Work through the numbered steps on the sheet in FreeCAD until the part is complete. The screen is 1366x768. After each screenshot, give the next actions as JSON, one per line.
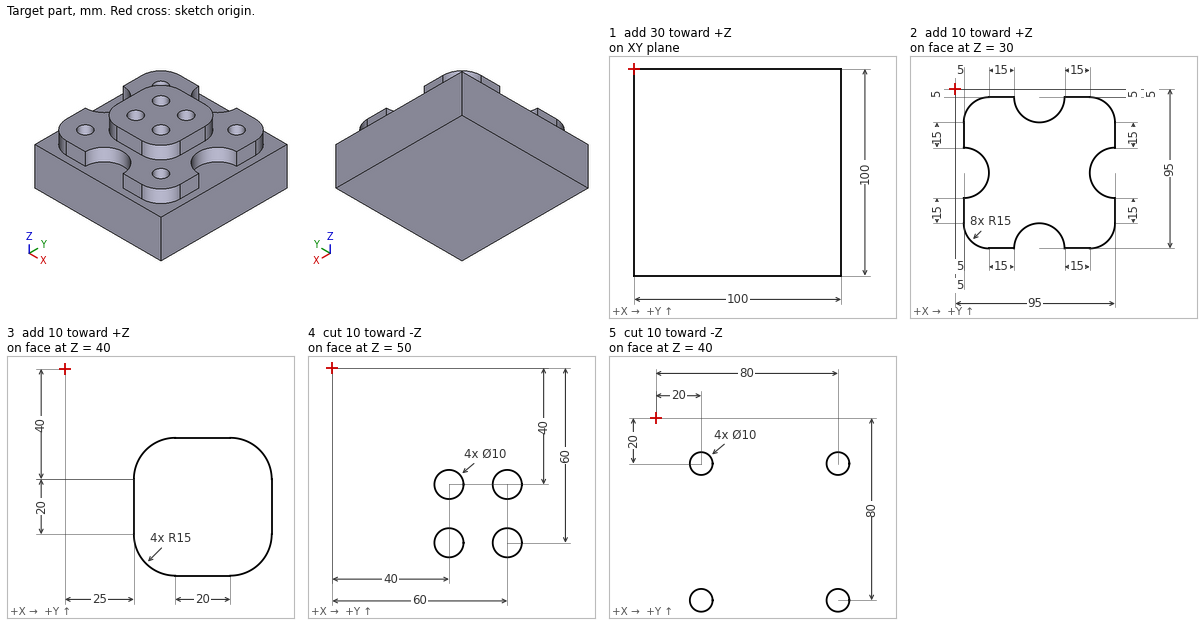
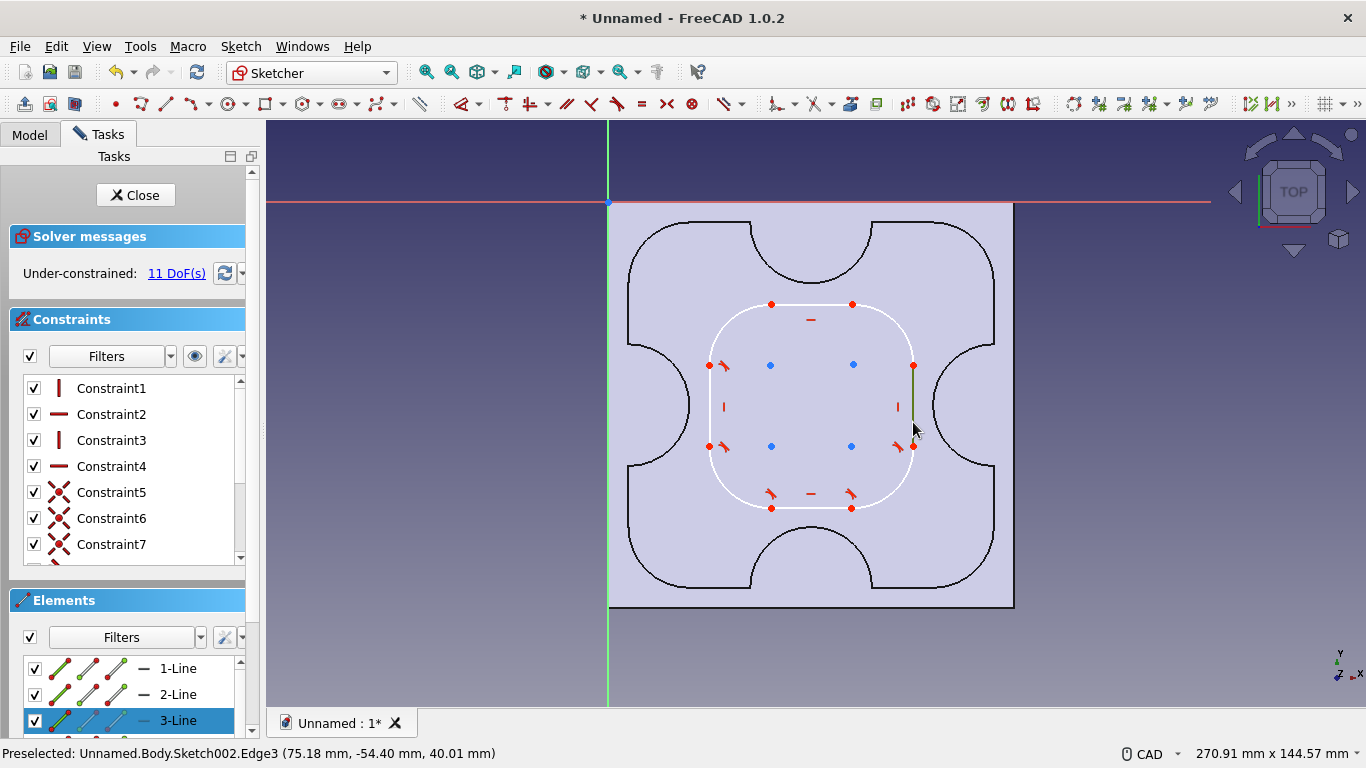
{"action": "left_click", "coordinate": [907, 338]}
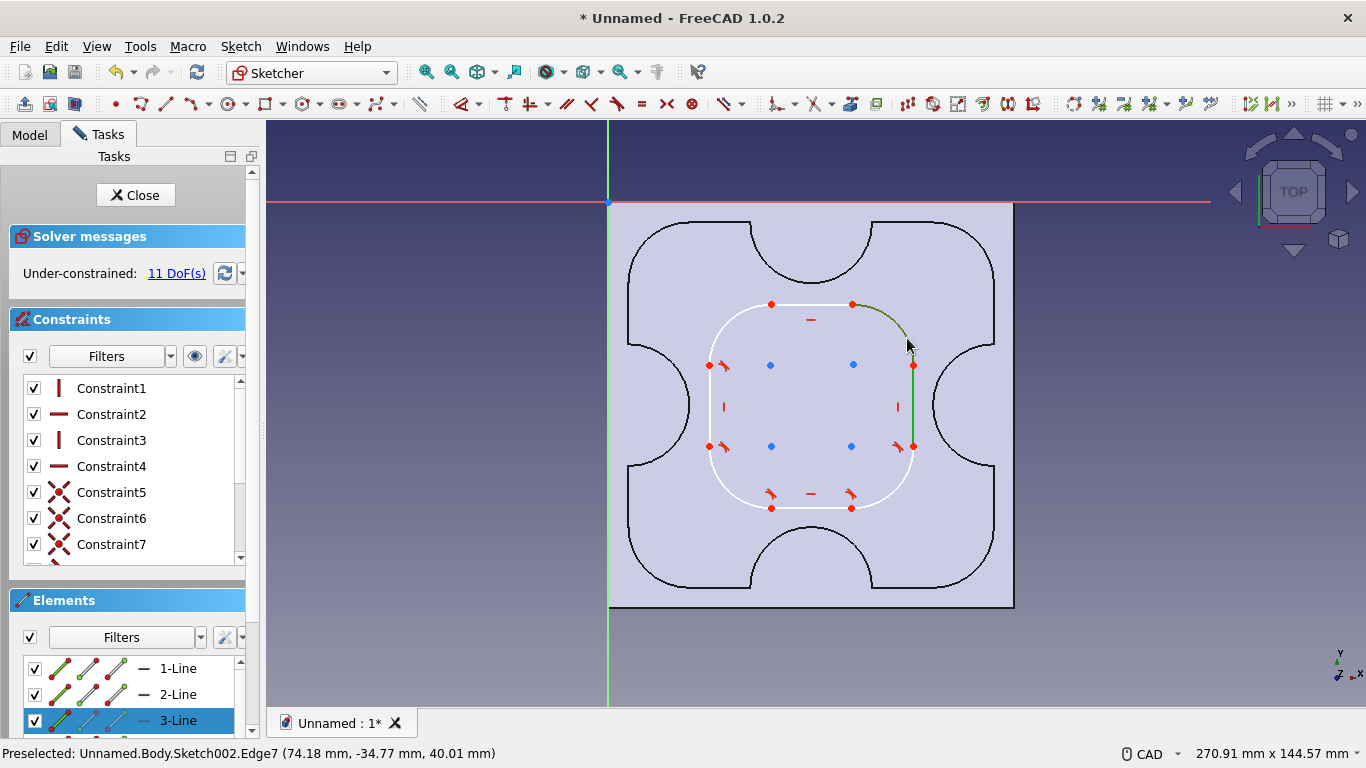
{"action": "key", "text": "t"}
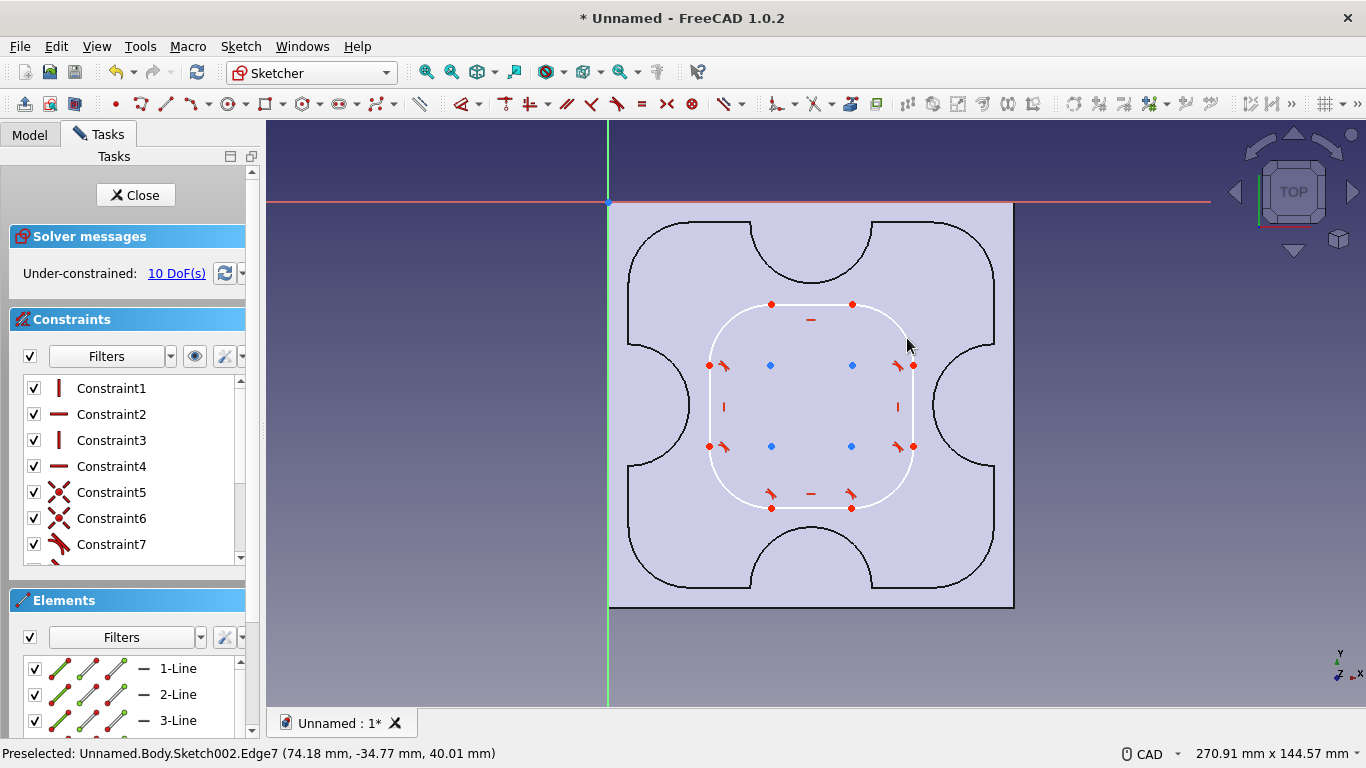
{"action": "left_click", "coordinate": [828, 305]}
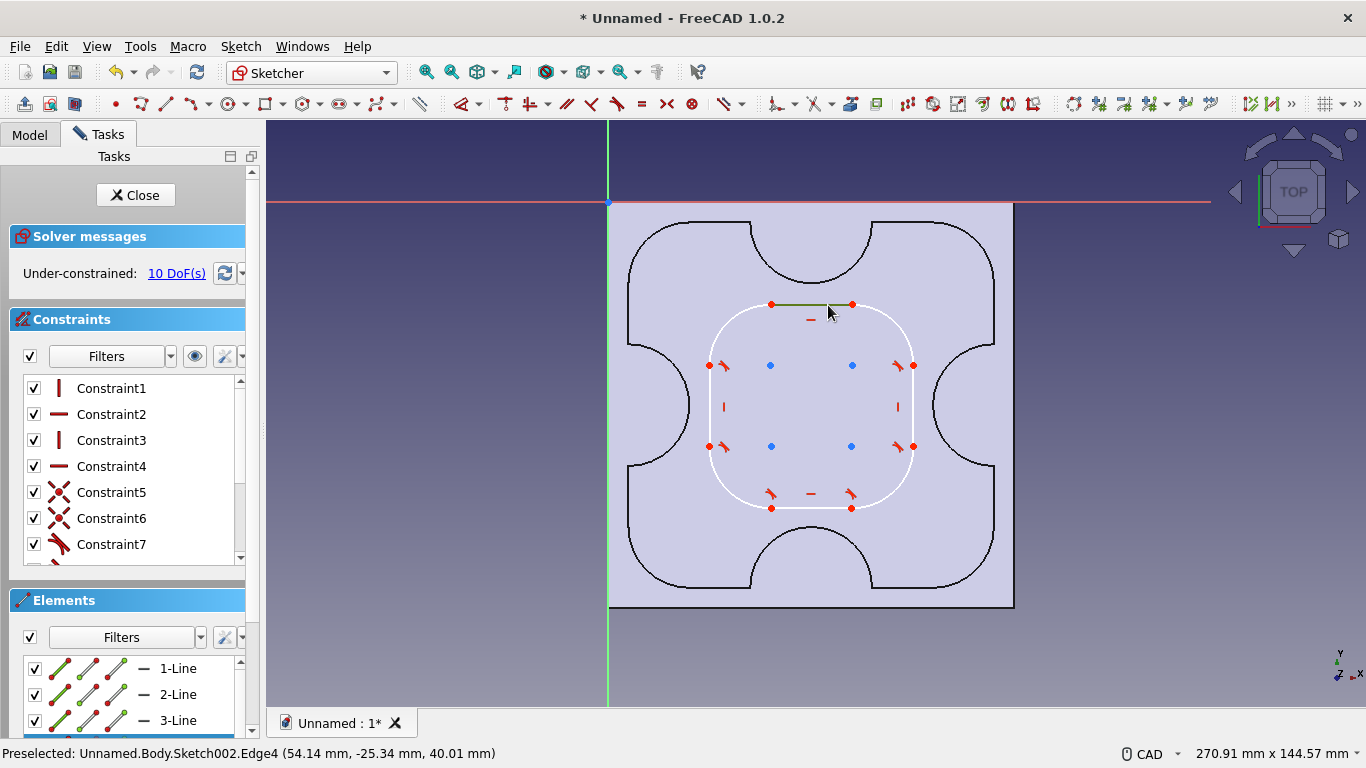
{"action": "left_click", "coordinate": [907, 338]}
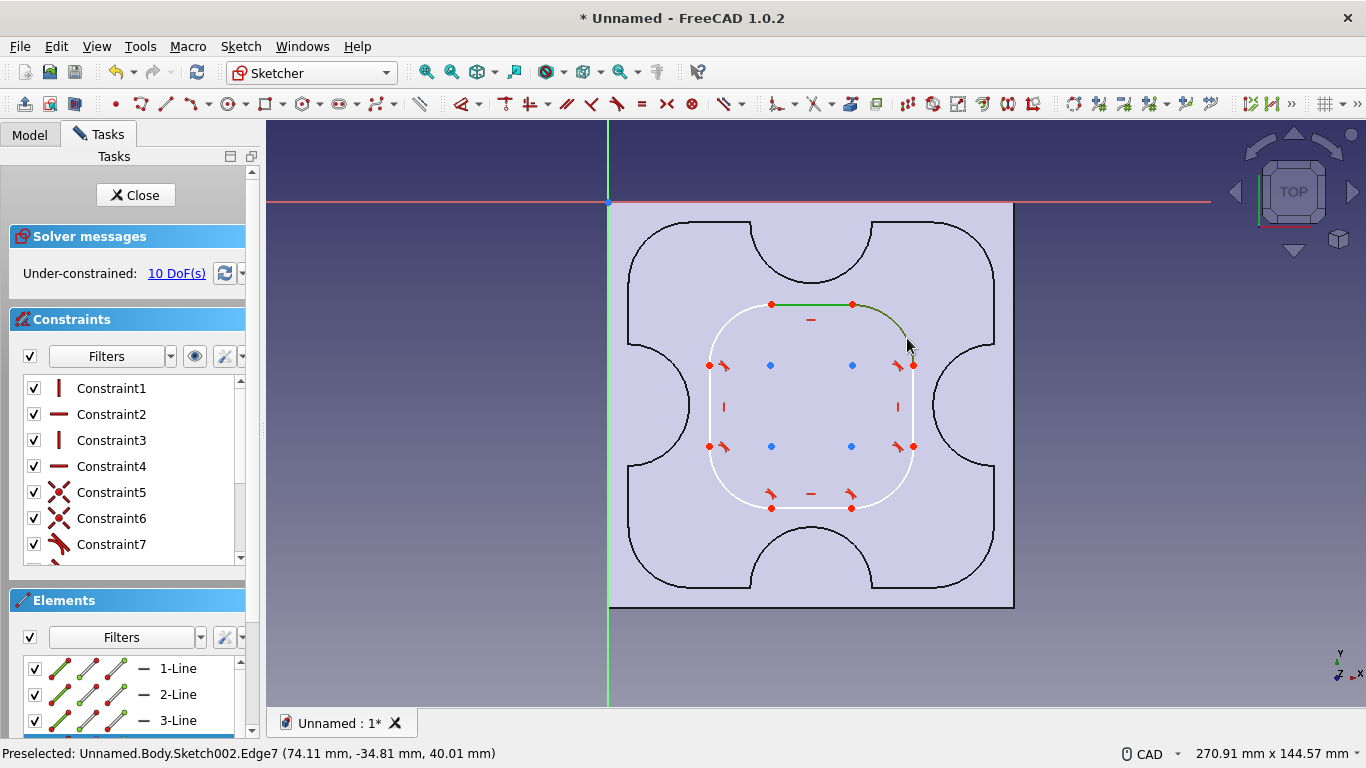
{"action": "left_click", "coordinate": [617, 104]}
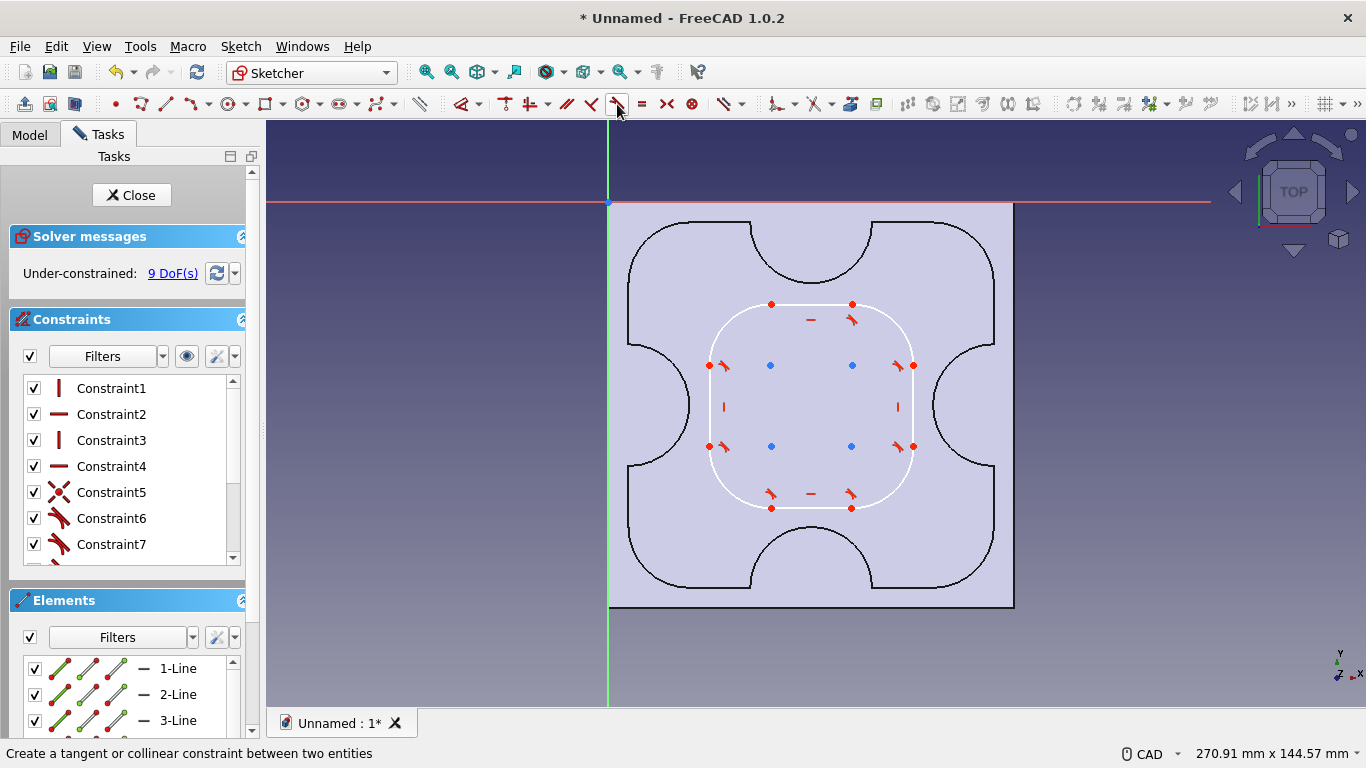
{"action": "left_click", "coordinate": [828, 305]}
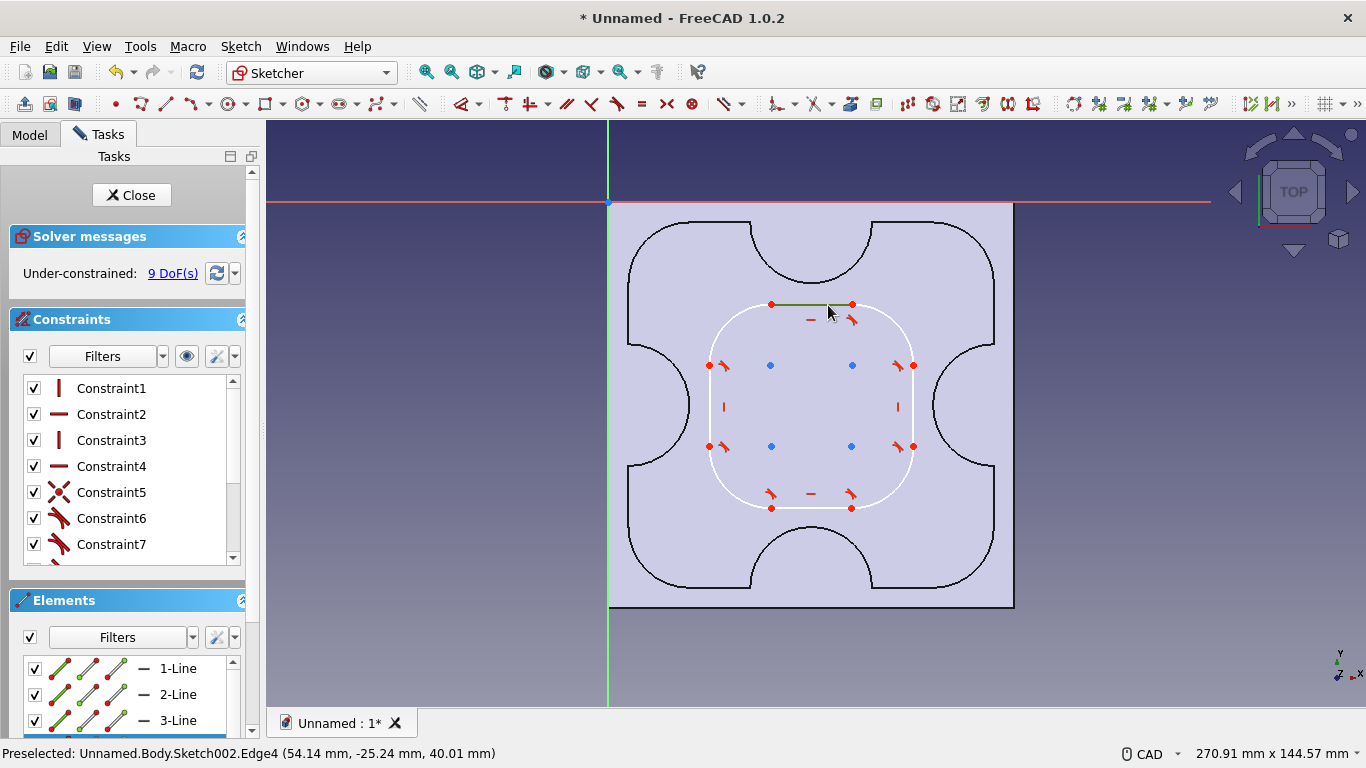
{"action": "left_click", "coordinate": [743, 311]}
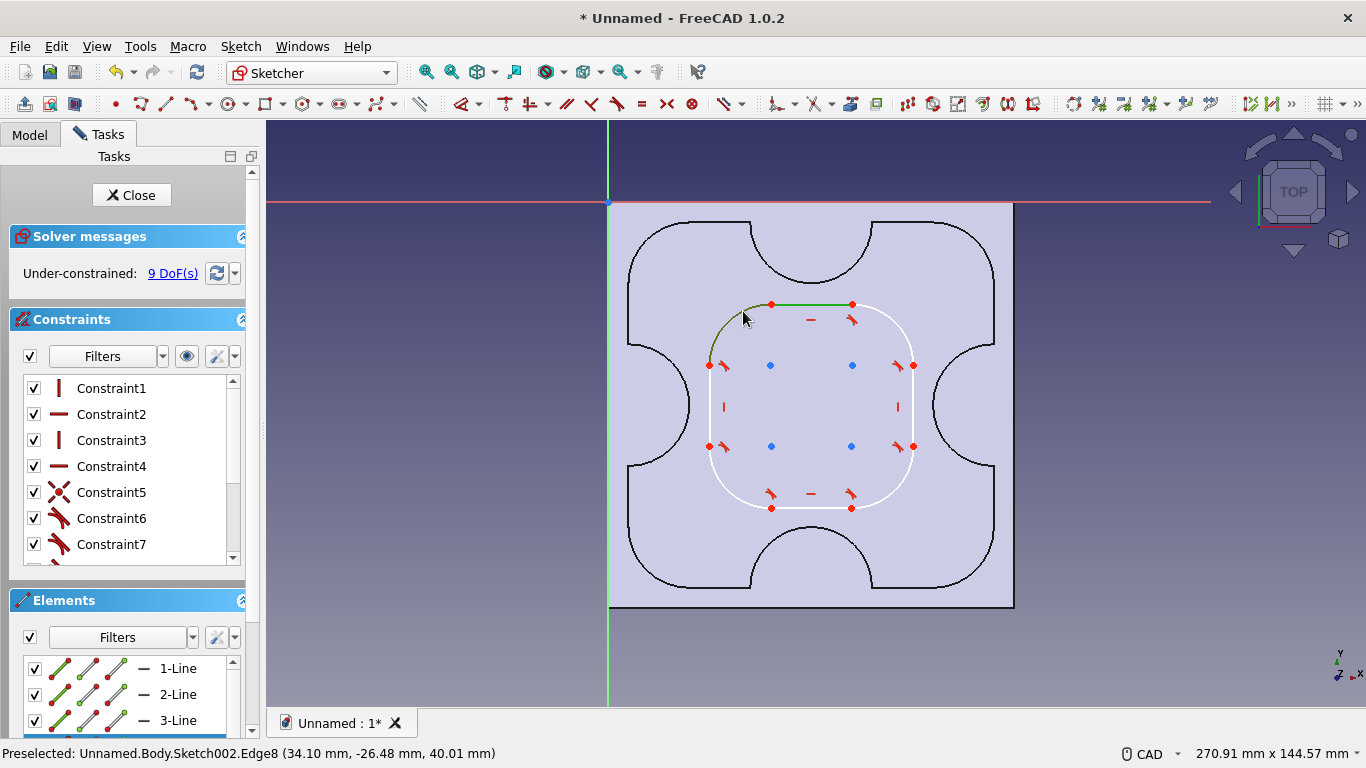
{"action": "left_click", "coordinate": [617, 104]}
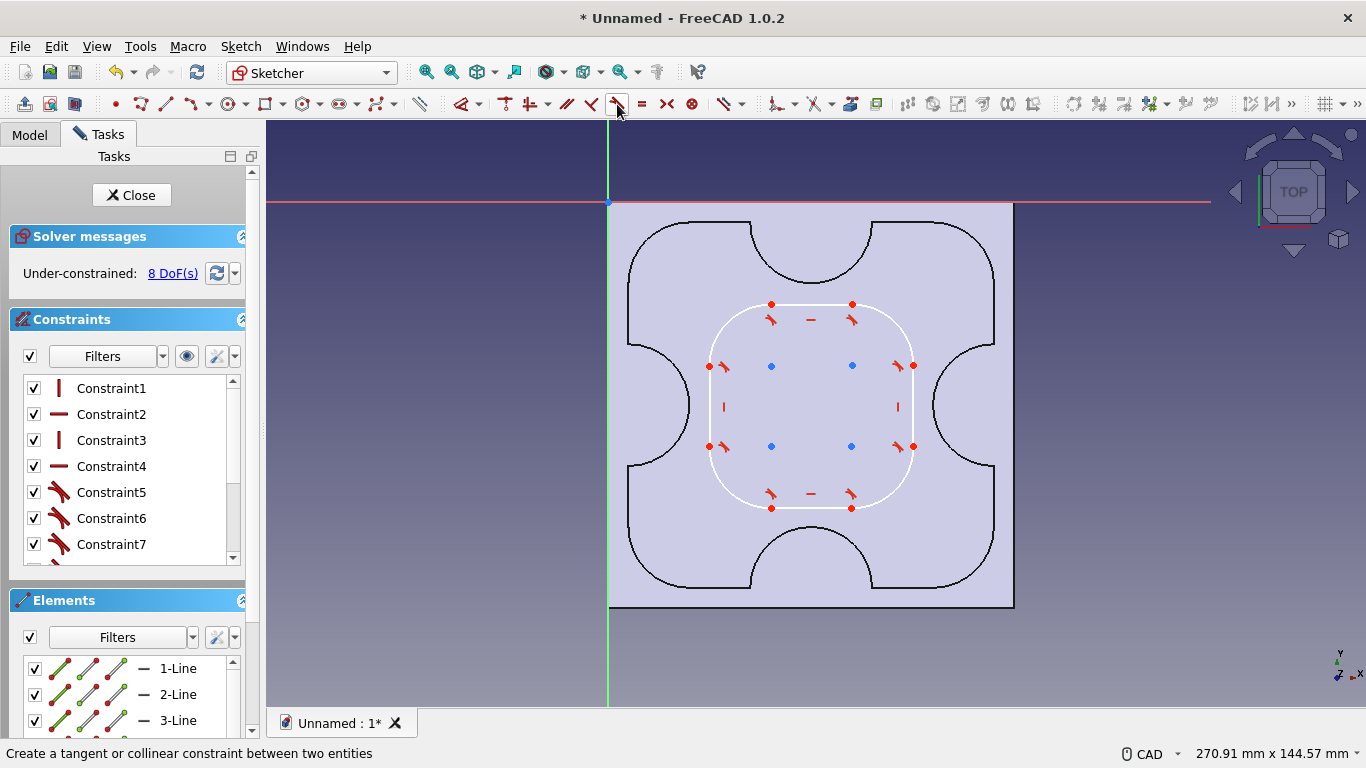
{"action": "left_click", "coordinate": [716, 475]}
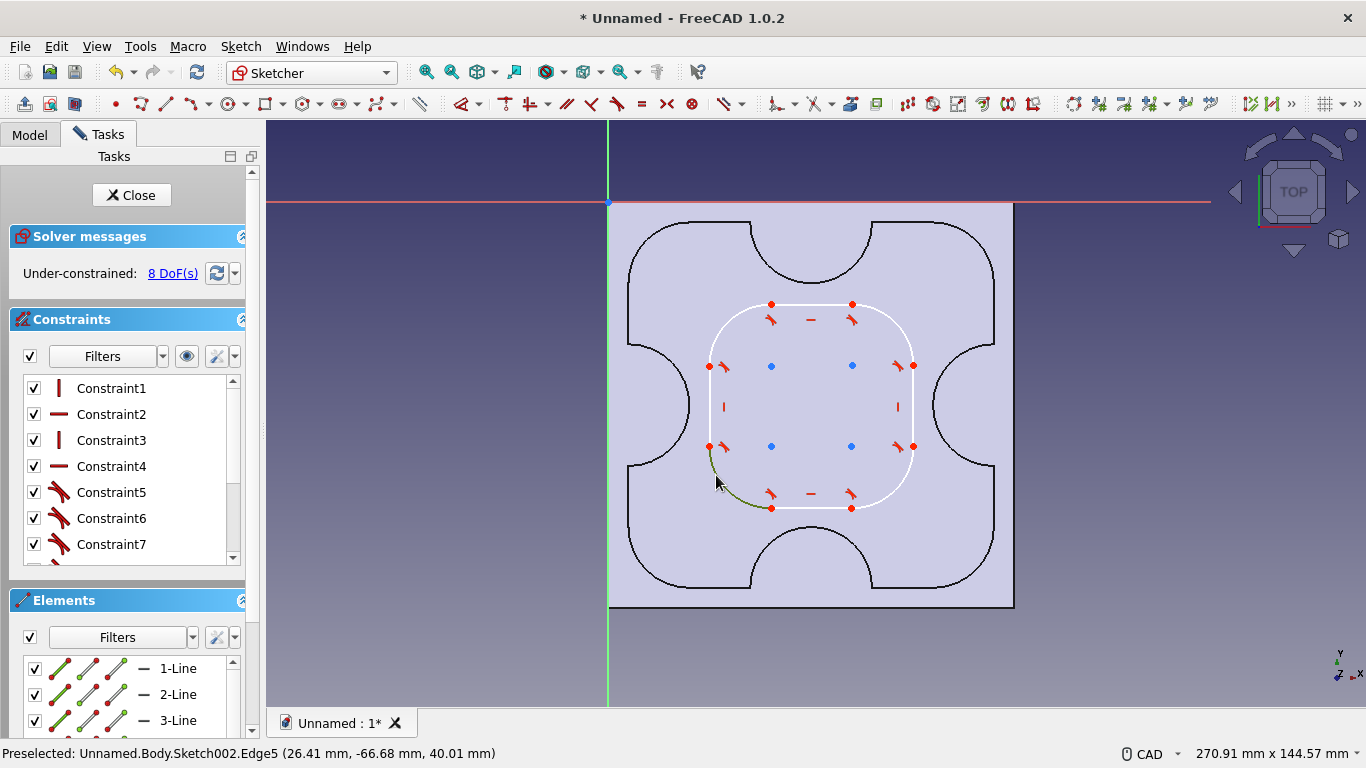
{"action": "left_click", "coordinate": [880, 501]}